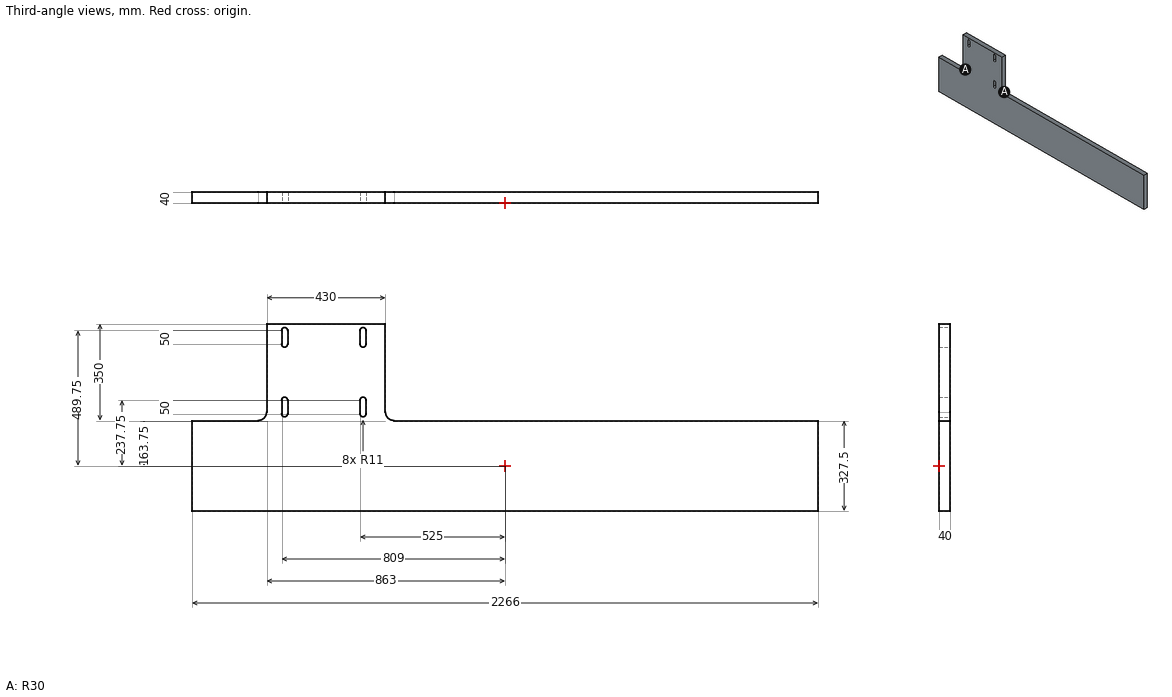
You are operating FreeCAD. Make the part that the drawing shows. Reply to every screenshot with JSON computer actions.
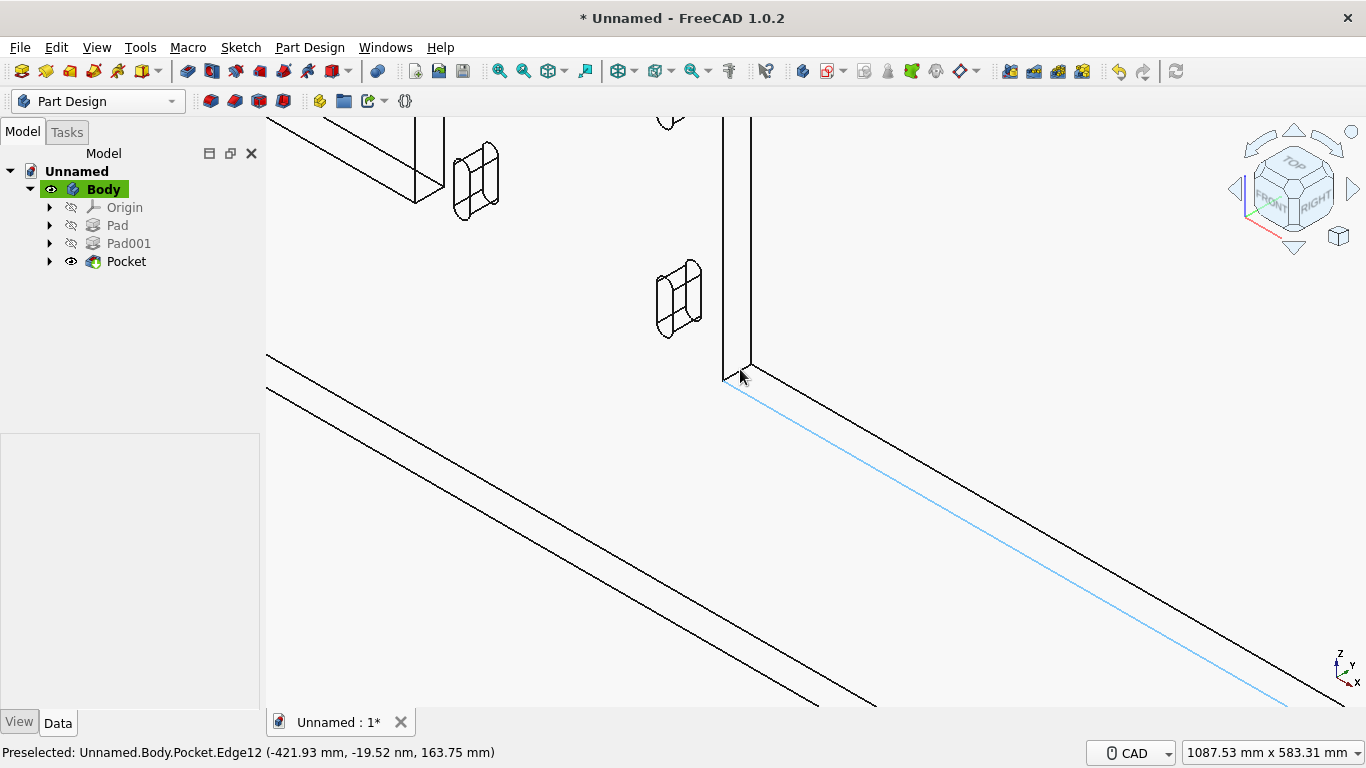
{"action": "left_click", "coordinate": [737, 372]}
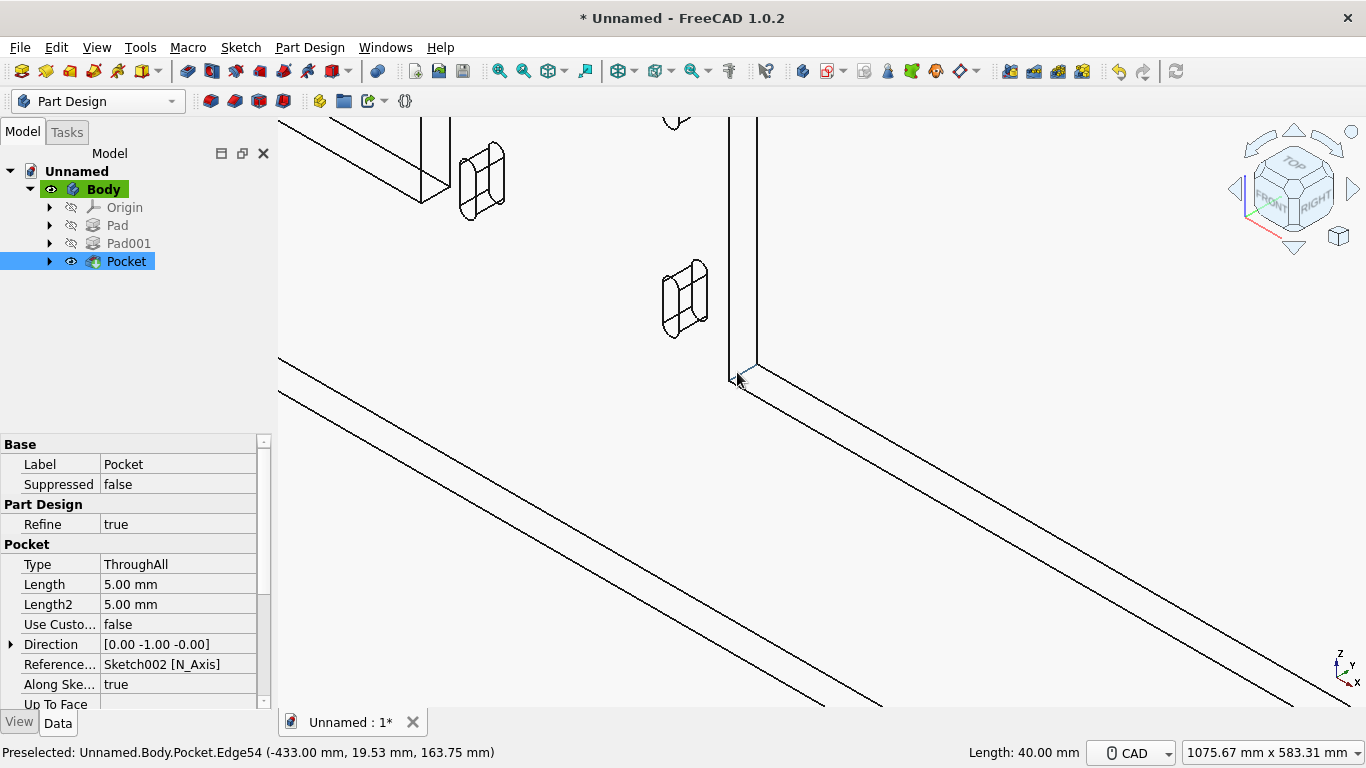
{"action": "left_click", "coordinate": [436, 194], "text": "ctrl"}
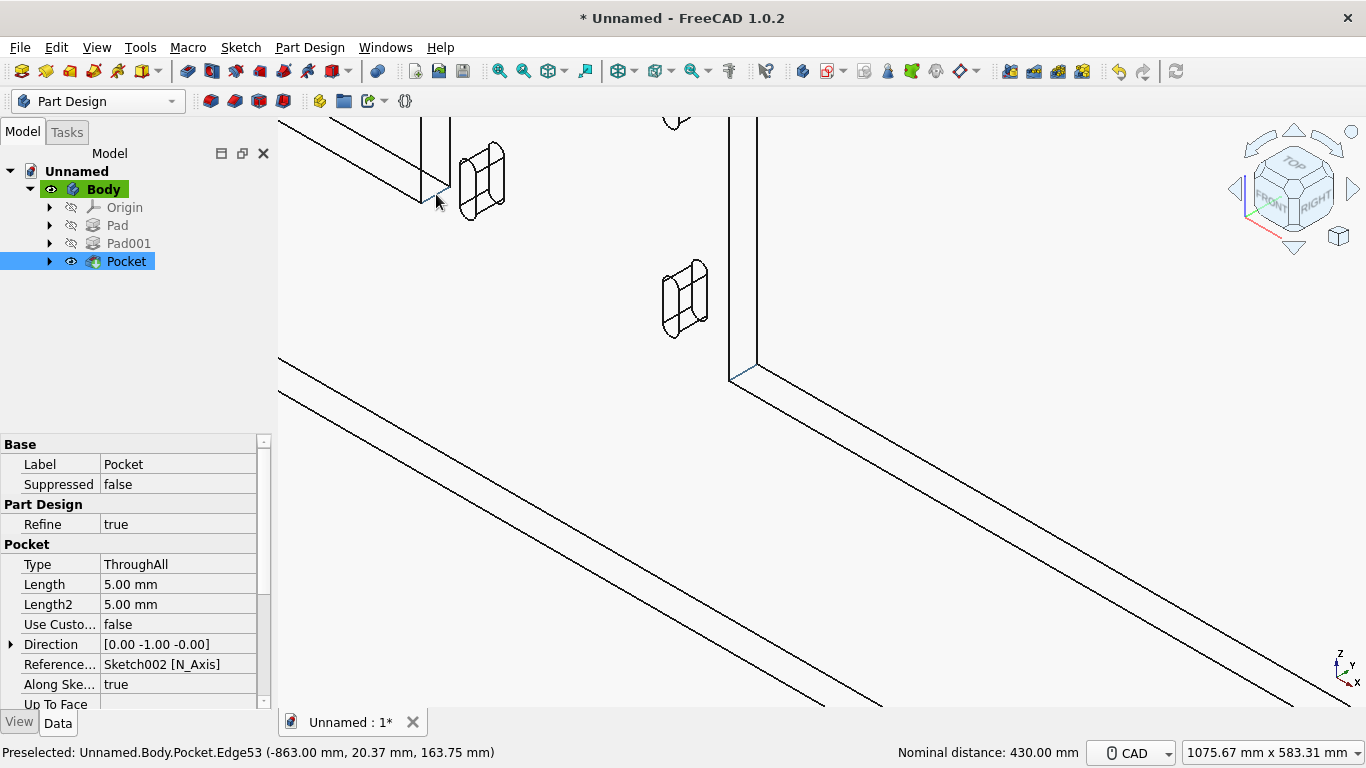
{"action": "key", "text": "v 1"}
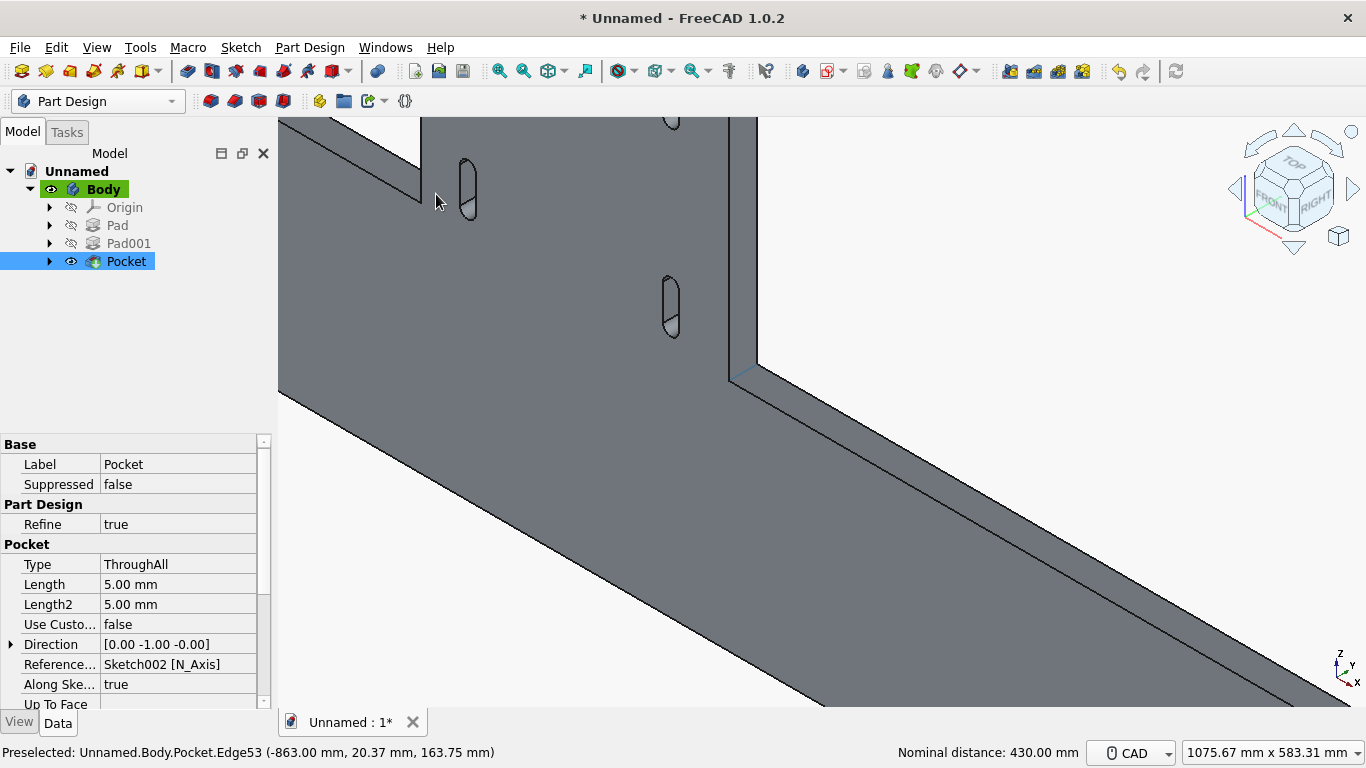
{"action": "left_click", "coordinate": [212, 102]}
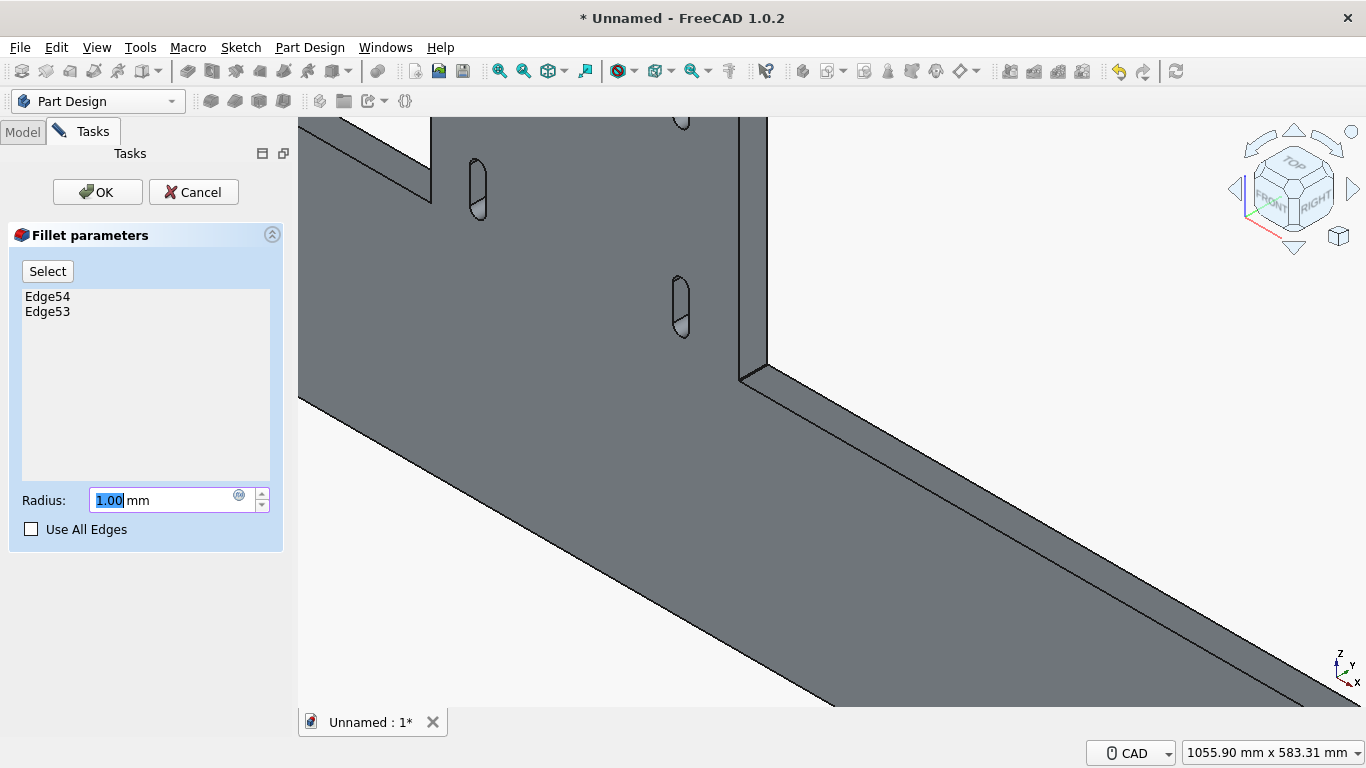
{"action": "type", "text": "30"}
{"action": "key", "text": "Tab"}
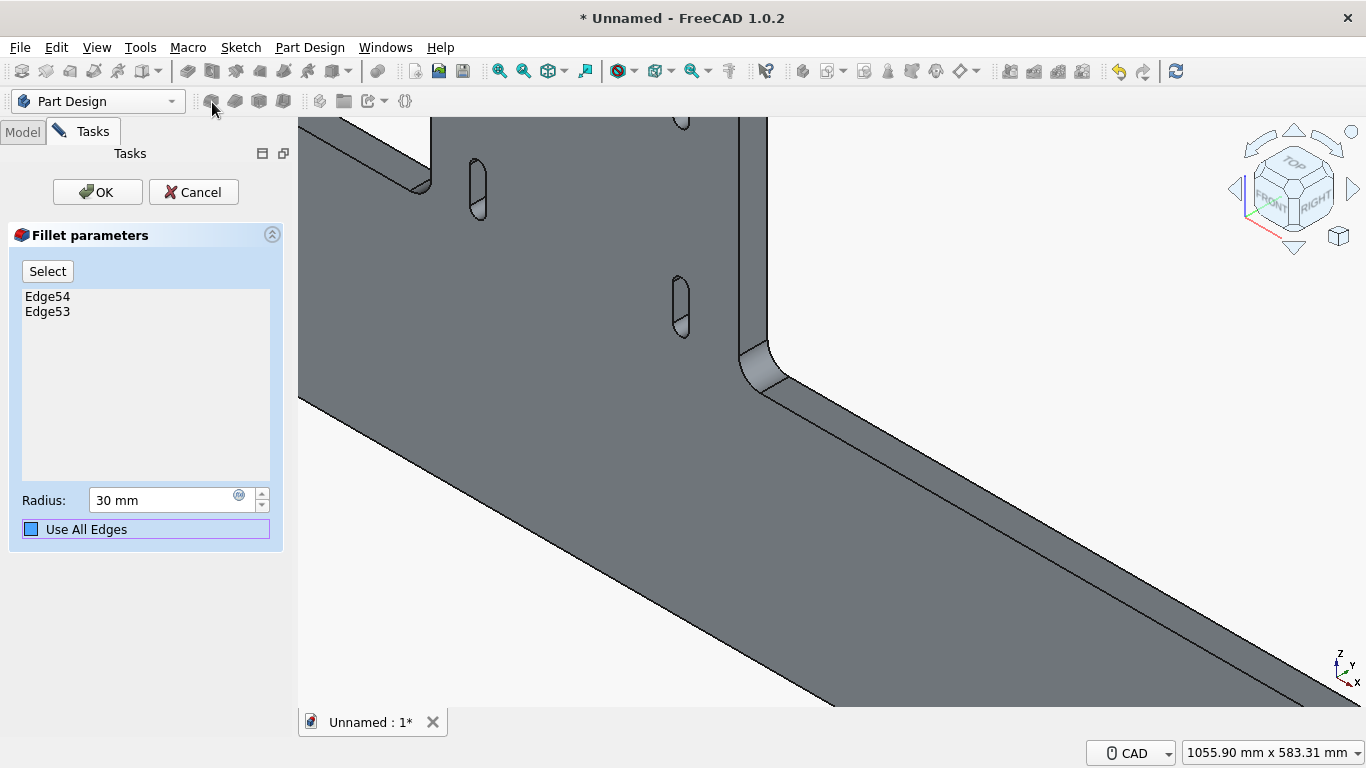
{"action": "left_click", "coordinate": [98, 192]}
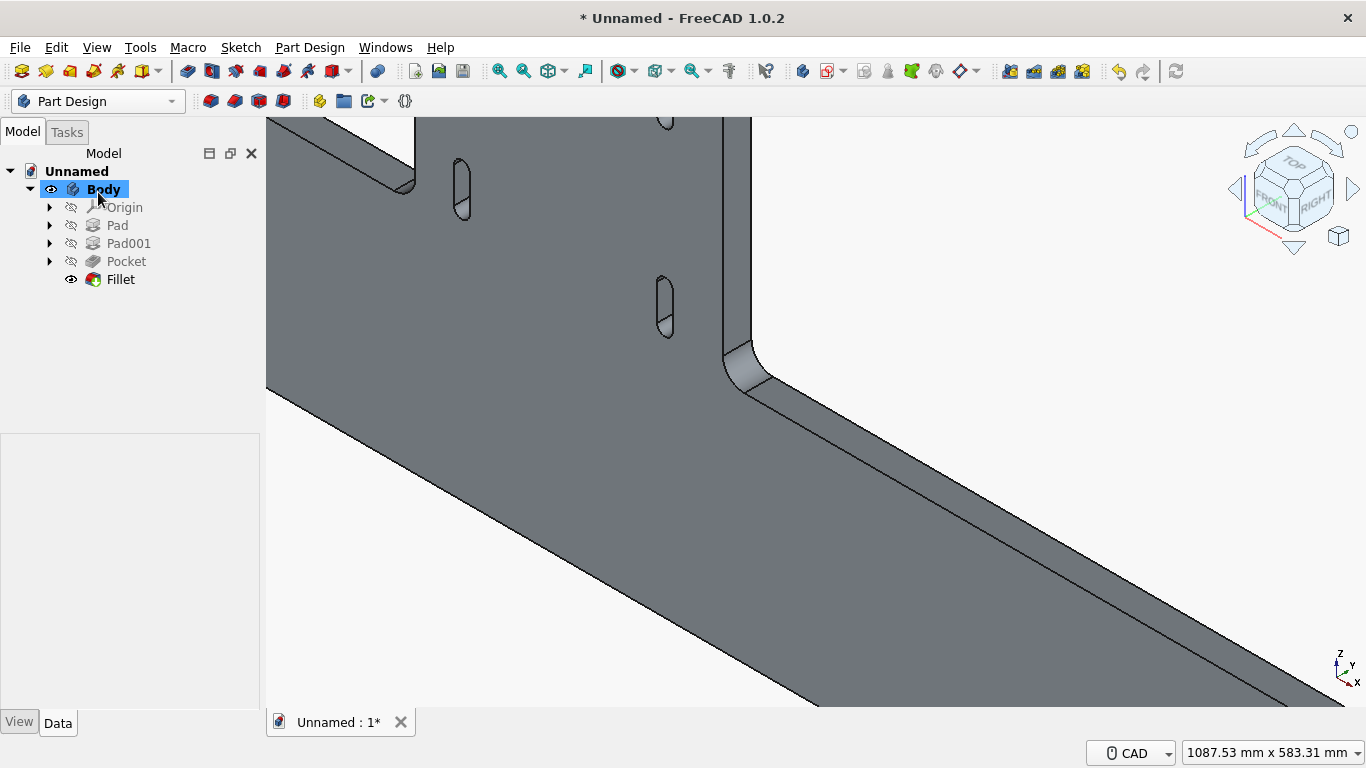
{"action": "left_click", "coordinate": [500, 72]}